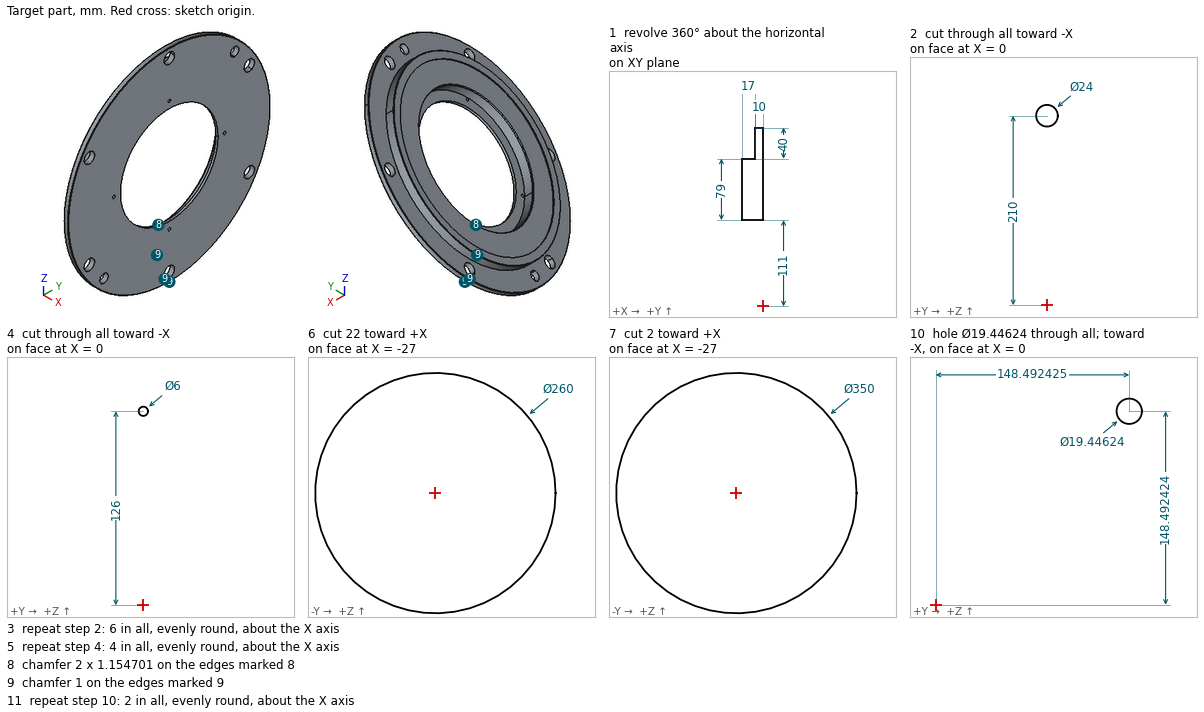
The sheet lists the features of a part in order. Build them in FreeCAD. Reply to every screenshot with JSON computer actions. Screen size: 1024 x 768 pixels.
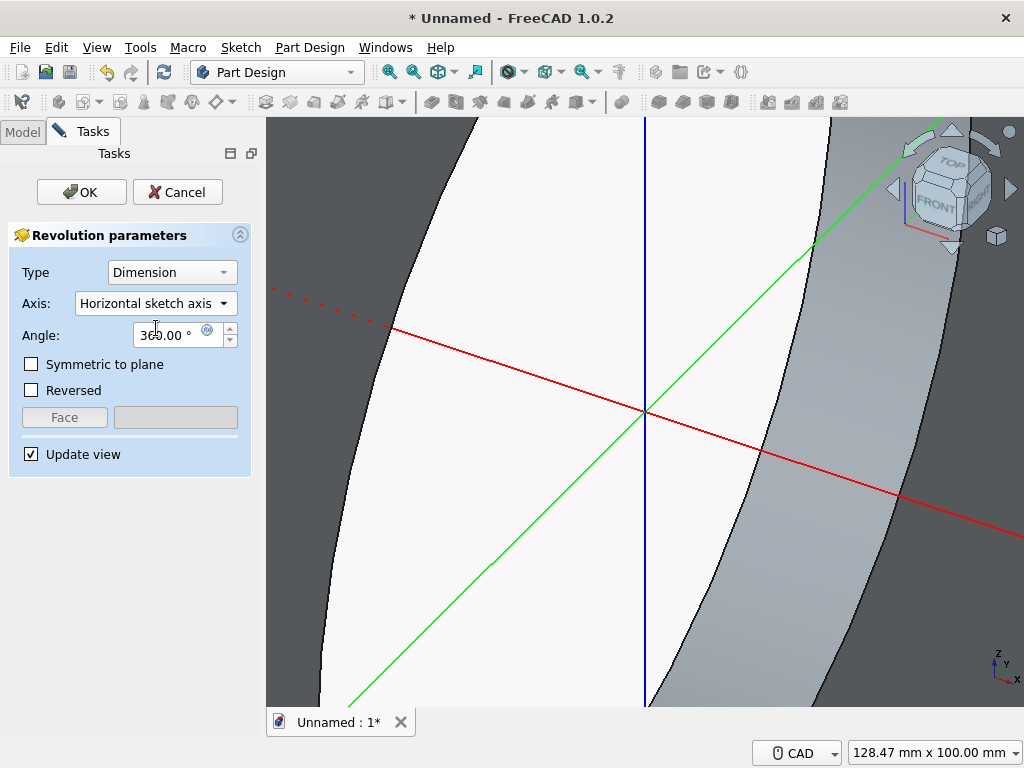
{"action": "left_click", "coordinate": [82, 192]}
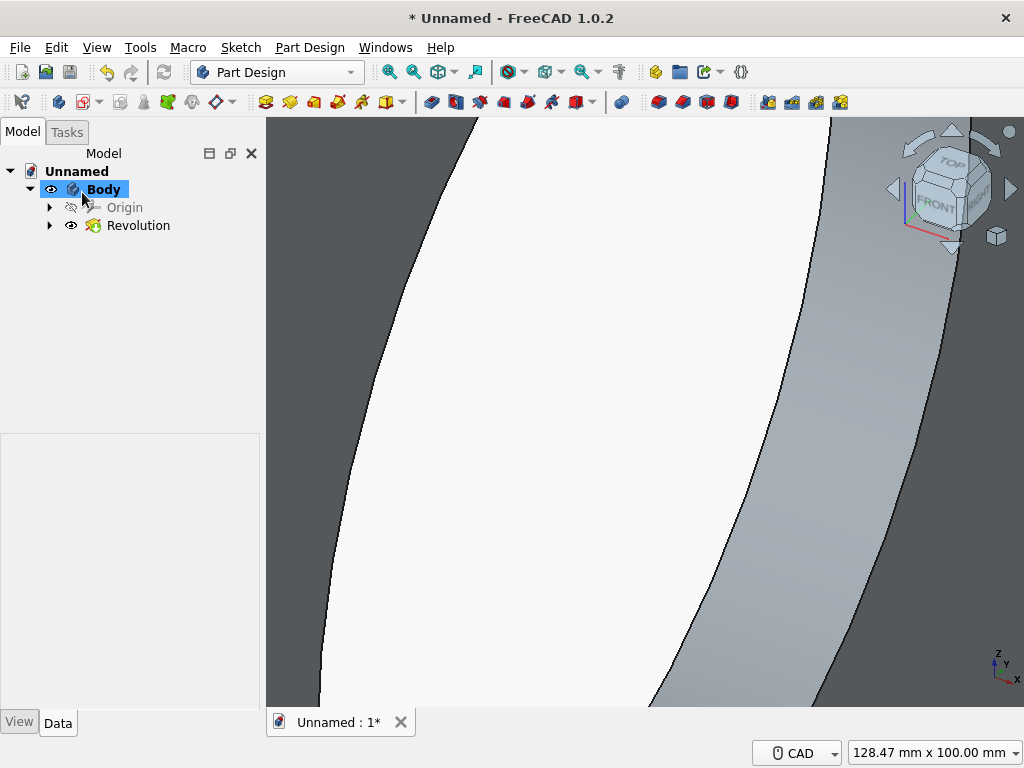
{"action": "key", "text": "v f"}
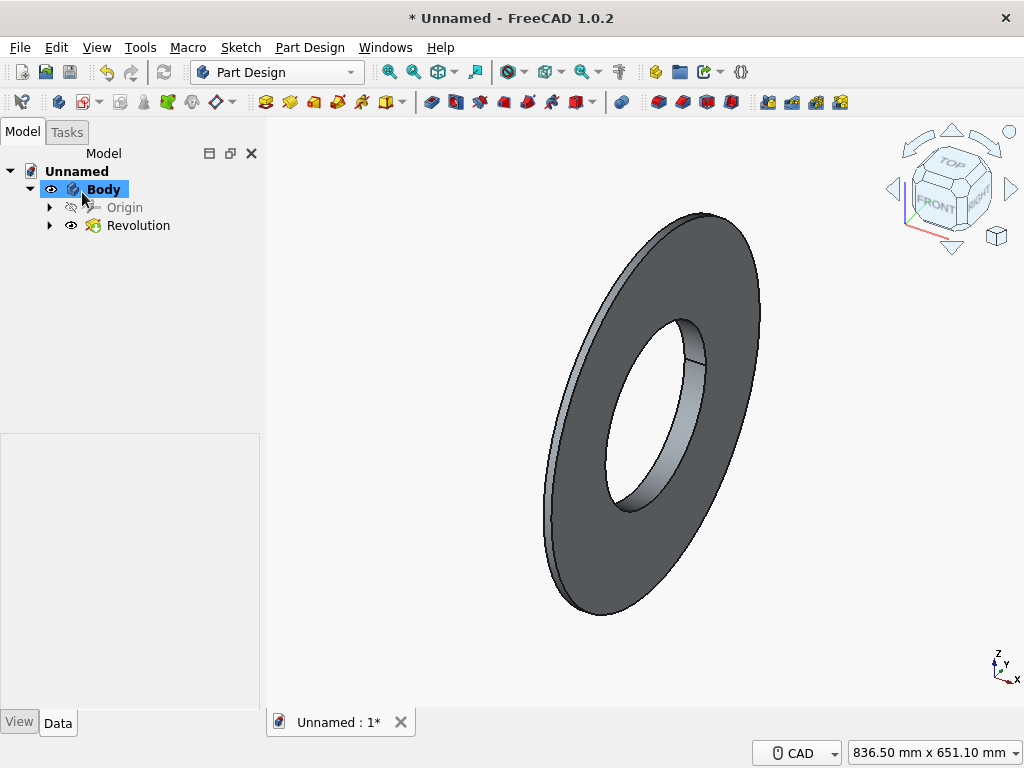
{"action": "left_click", "coordinate": [596, 571]}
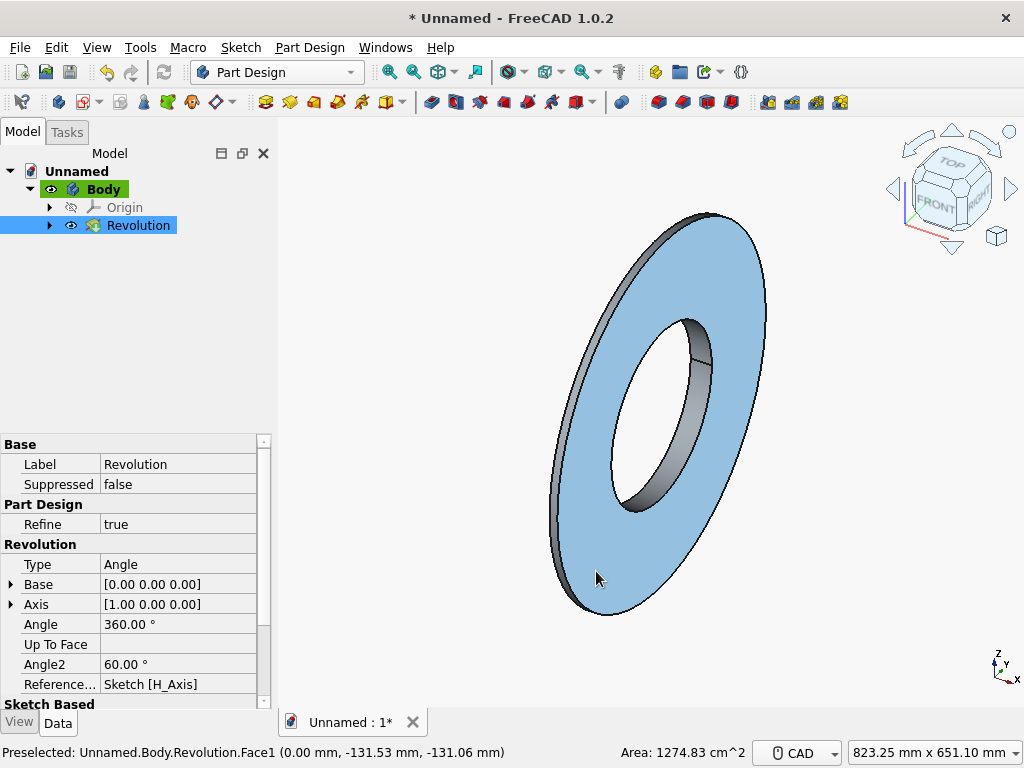
{"action": "left_click", "coordinate": [84, 102]}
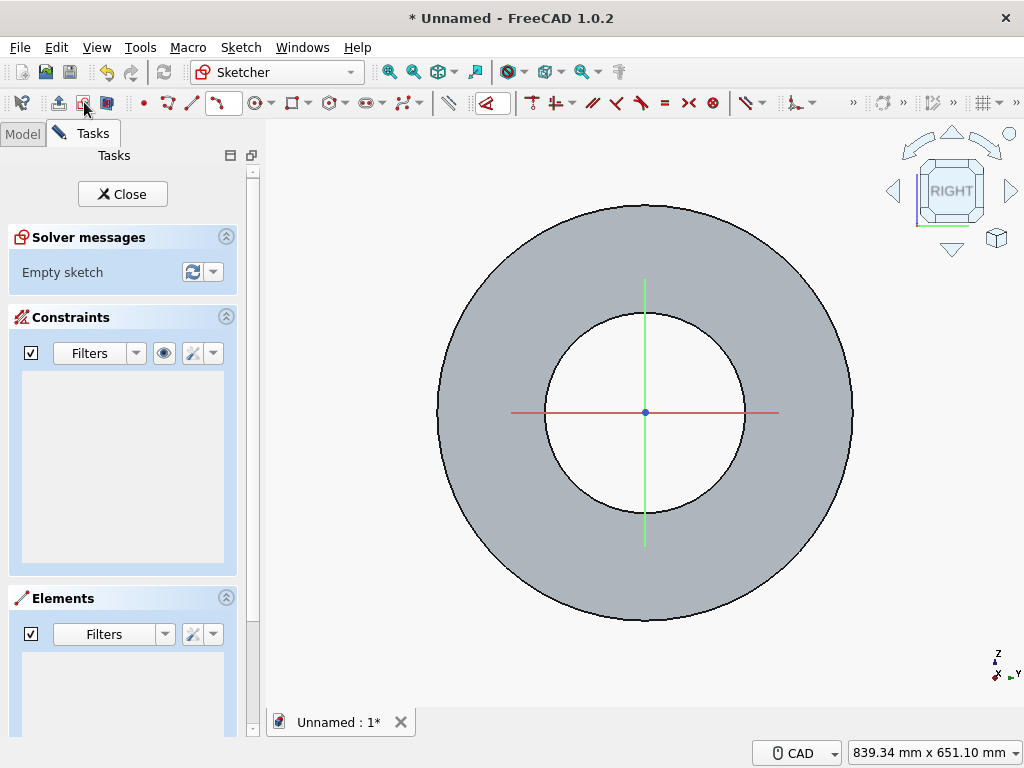
{"action": "scroll", "coordinate": [649, 211], "scroll_direction": "up", "scroll_amount": 14}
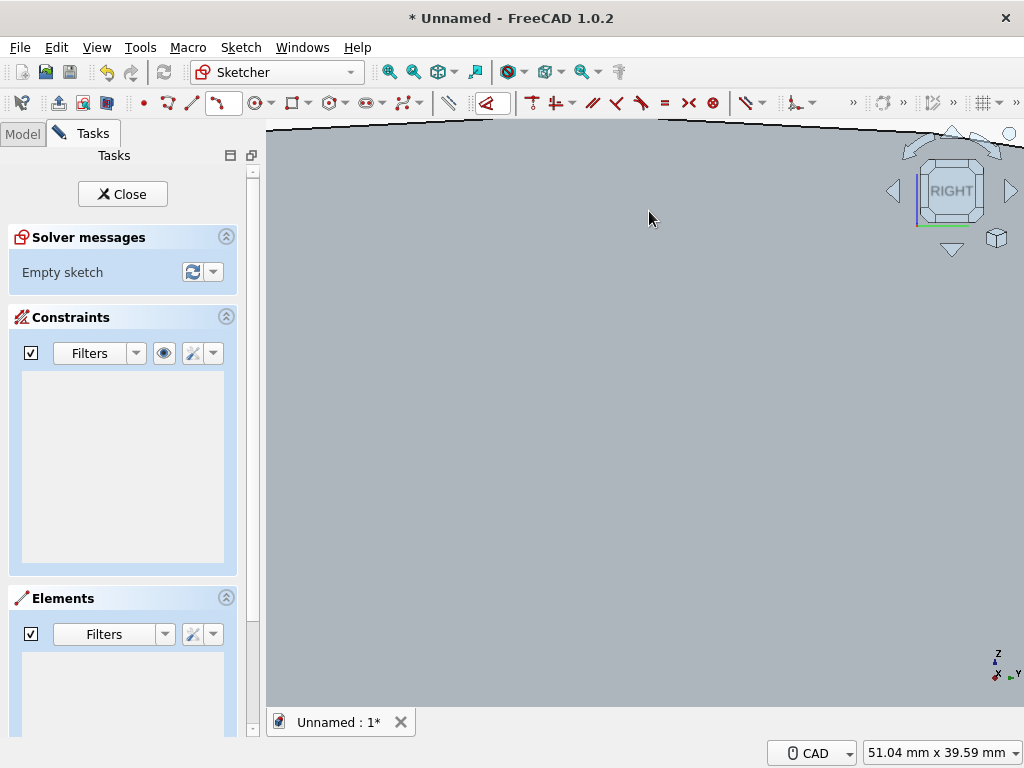
{"action": "key", "text": "g c"}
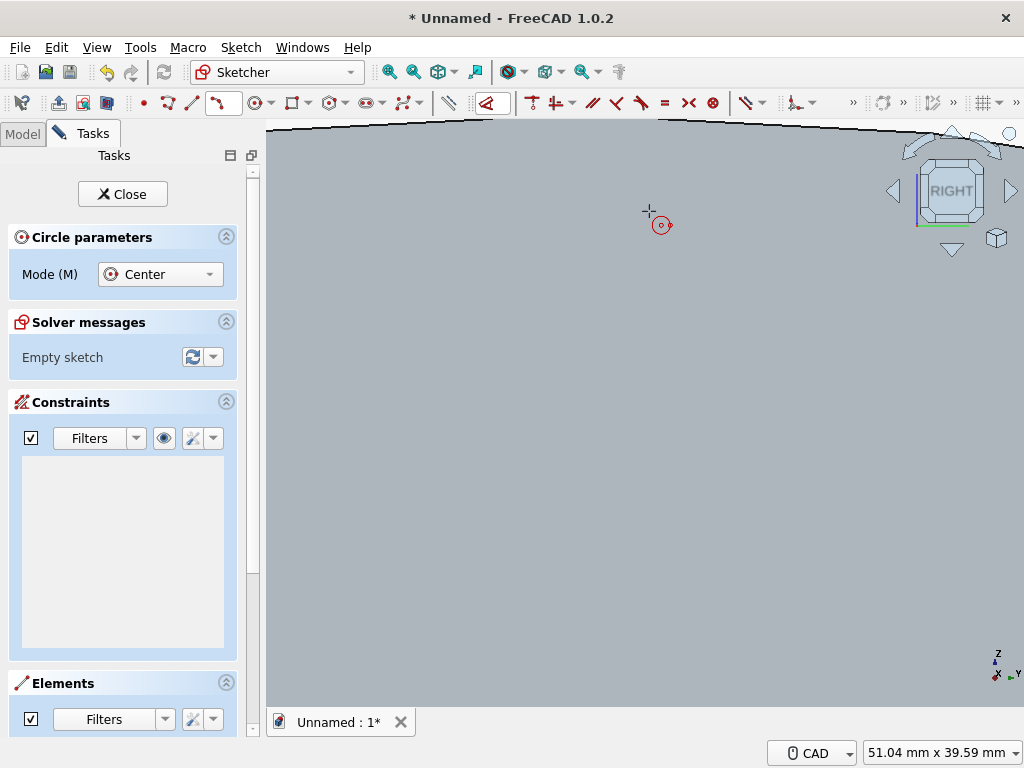
{"action": "left_click", "coordinate": [575, 412]}
{"action": "mouse_move", "coordinate": [701, 286]}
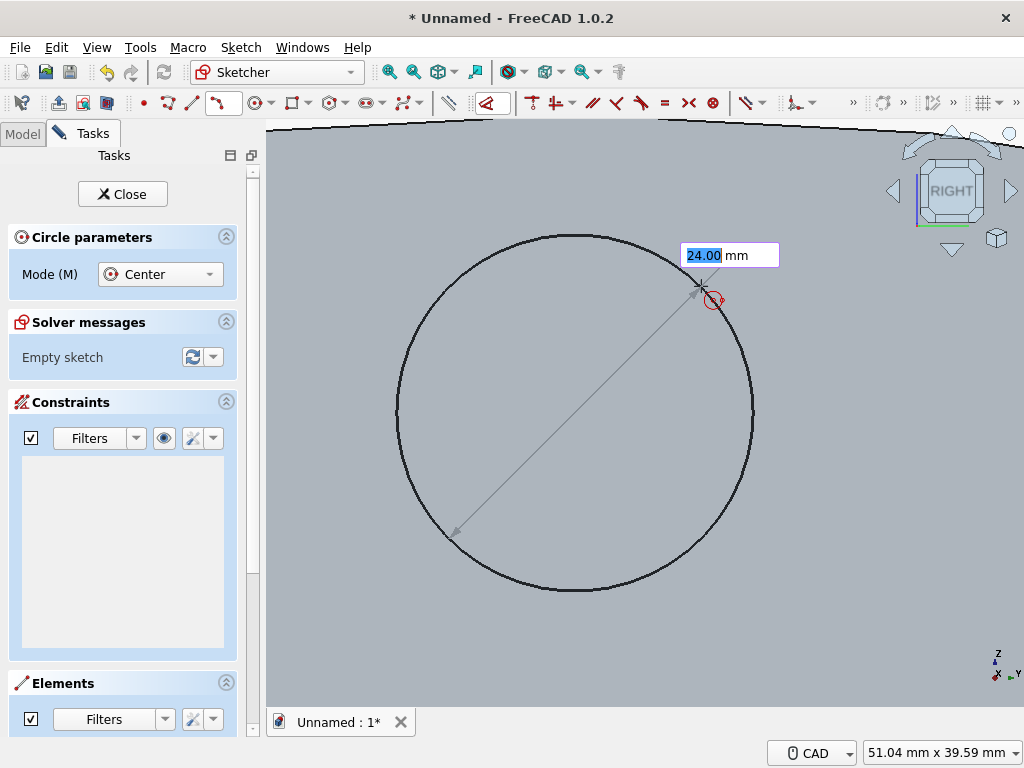
{"action": "type", "text": "24"}
{"action": "key", "text": "Return"}
{"action": "key", "text": "Escape"}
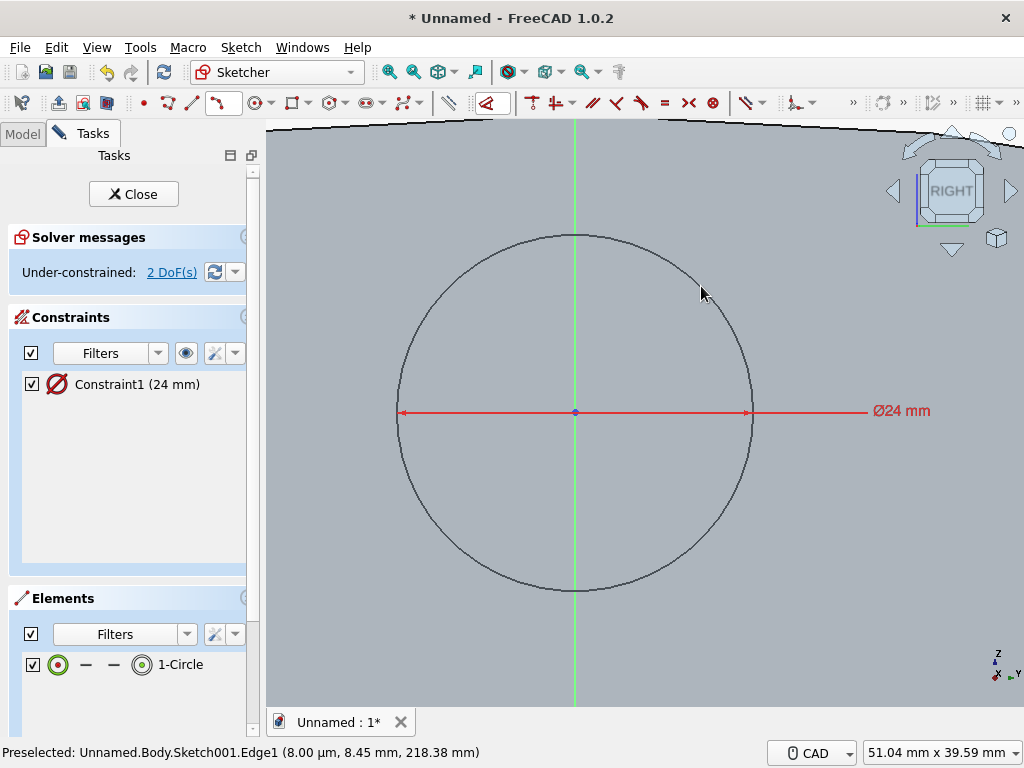
{"action": "left_click", "coordinate": [575, 413]}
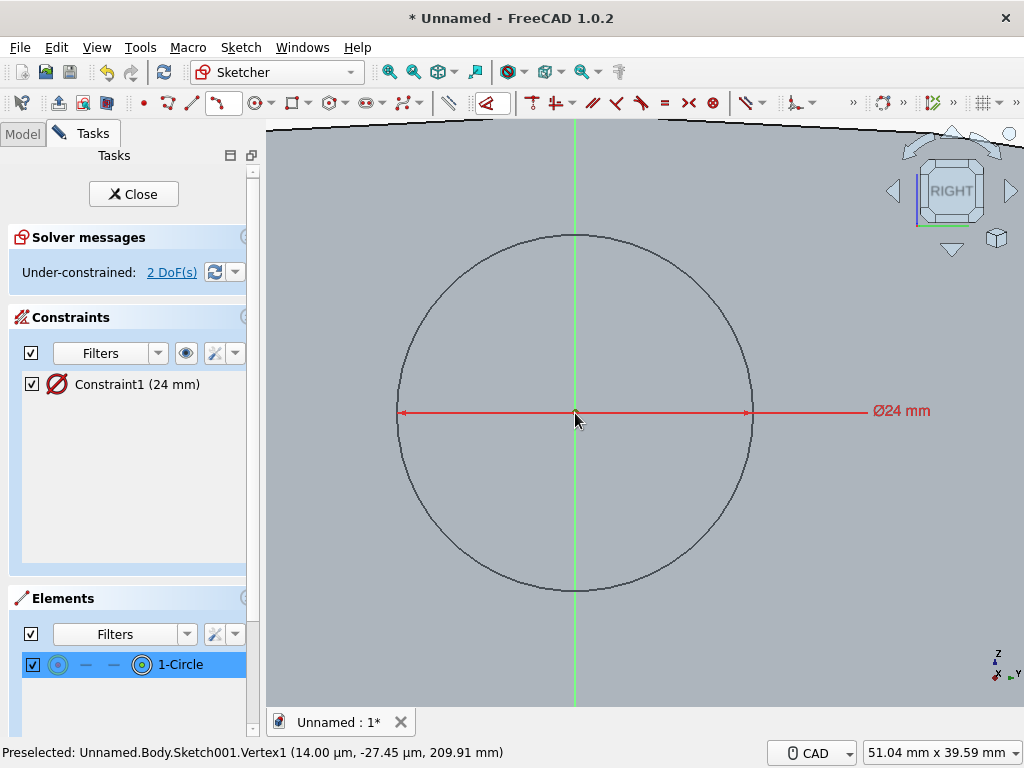
{"action": "left_click", "coordinate": [575, 641]}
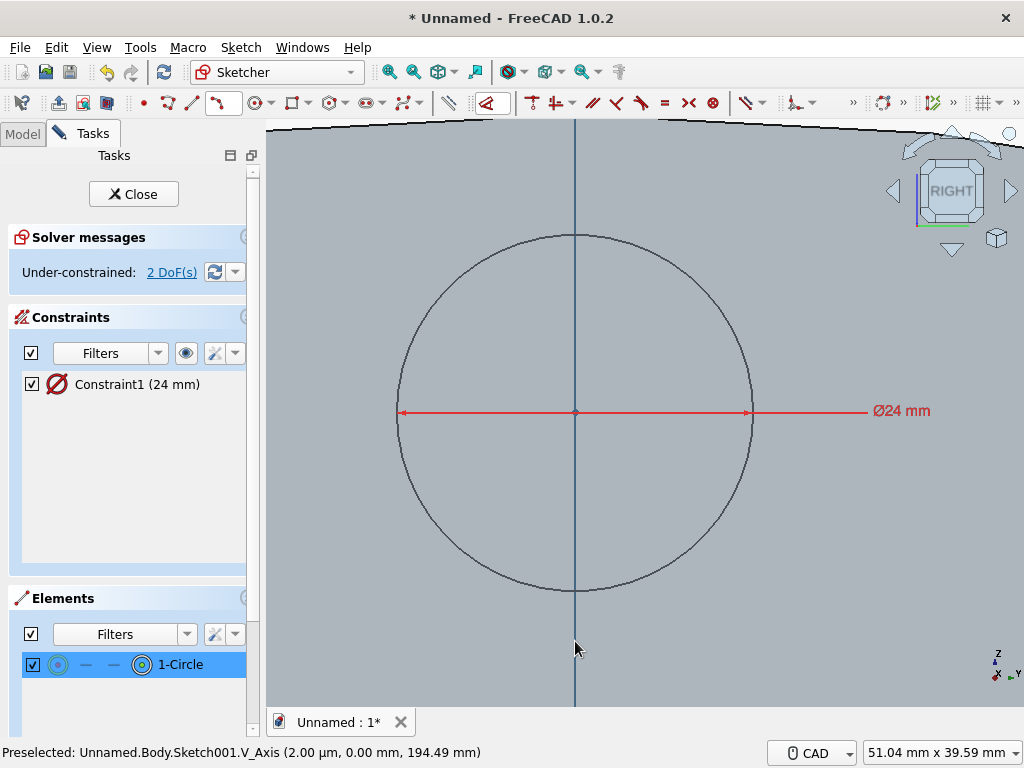
{"action": "key", "text": "c"}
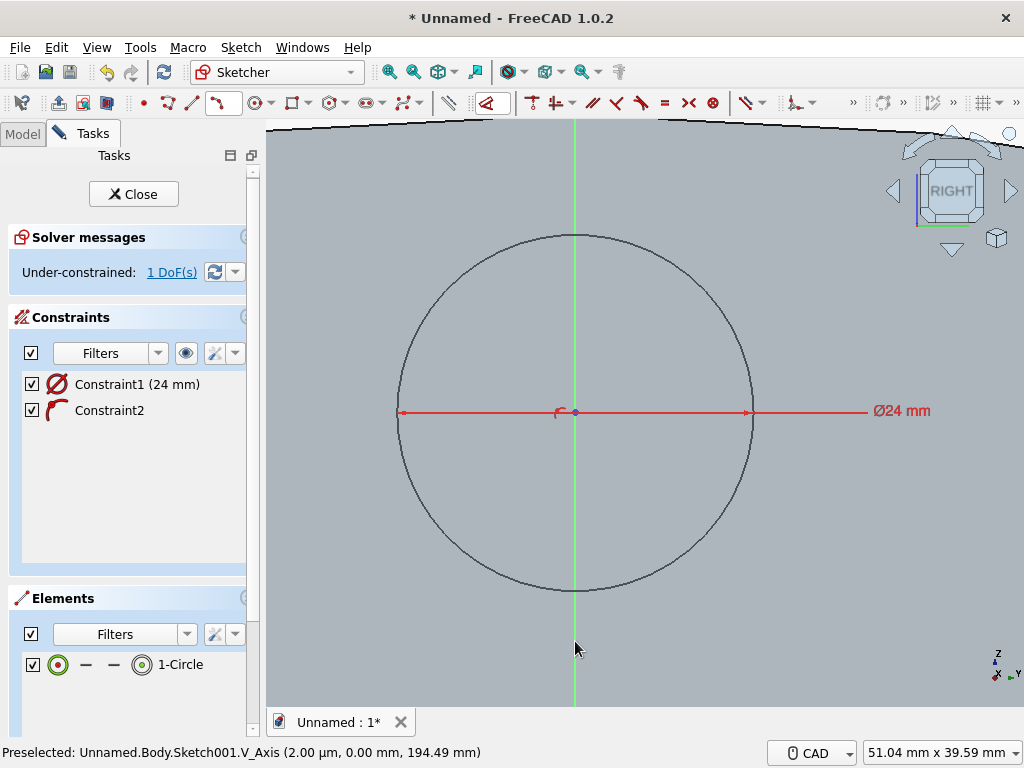
{"action": "key", "text": "d"}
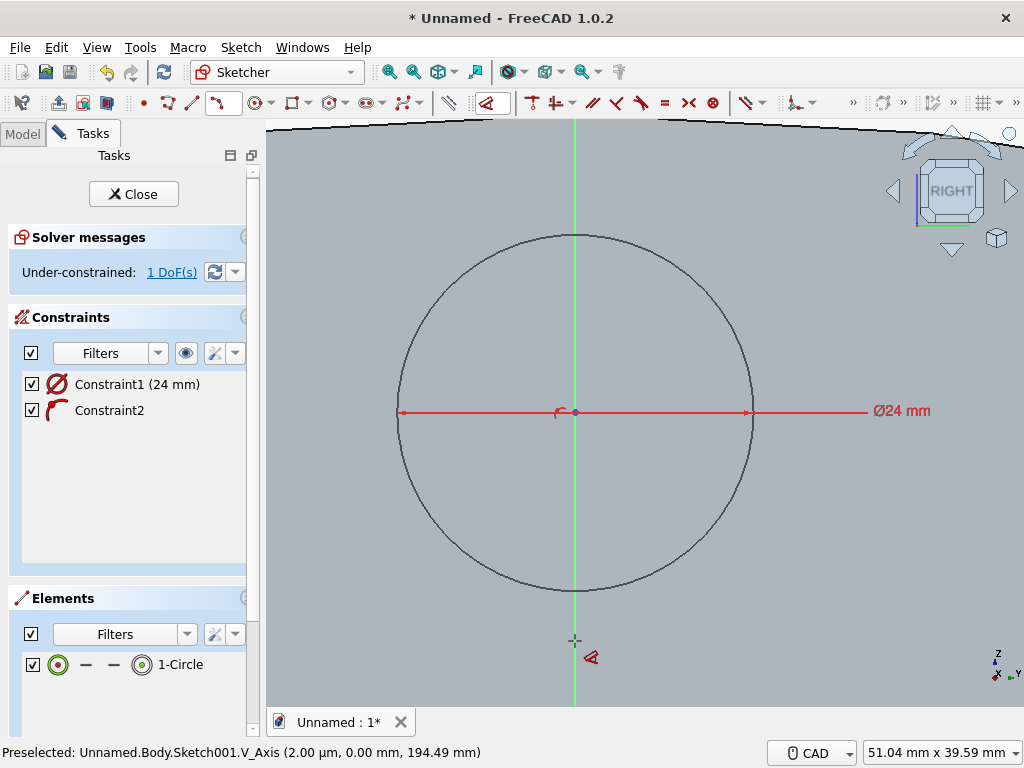
{"action": "left_click", "coordinate": [575, 413]}
{"action": "left_click", "coordinate": [609, 546]}